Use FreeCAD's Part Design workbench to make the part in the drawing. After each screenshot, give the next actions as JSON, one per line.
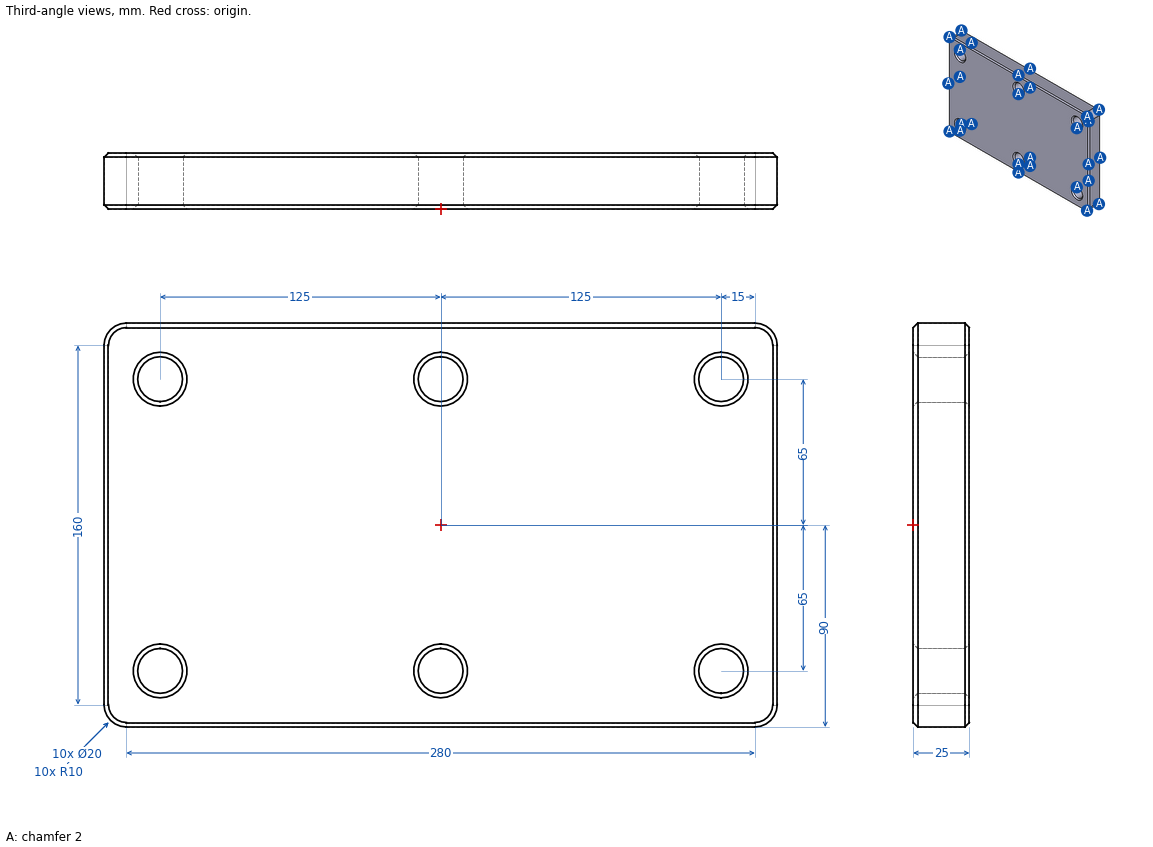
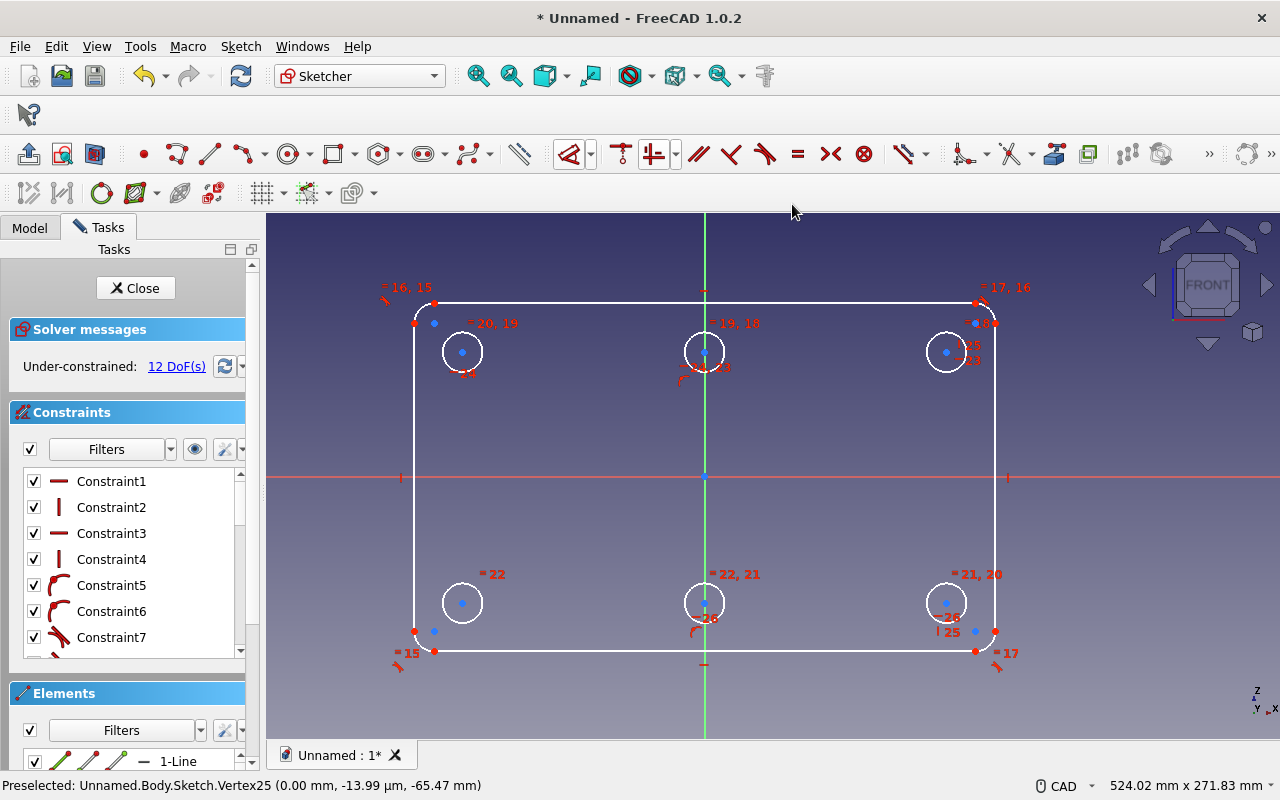
{"action": "left_click", "coordinate": [463, 352]}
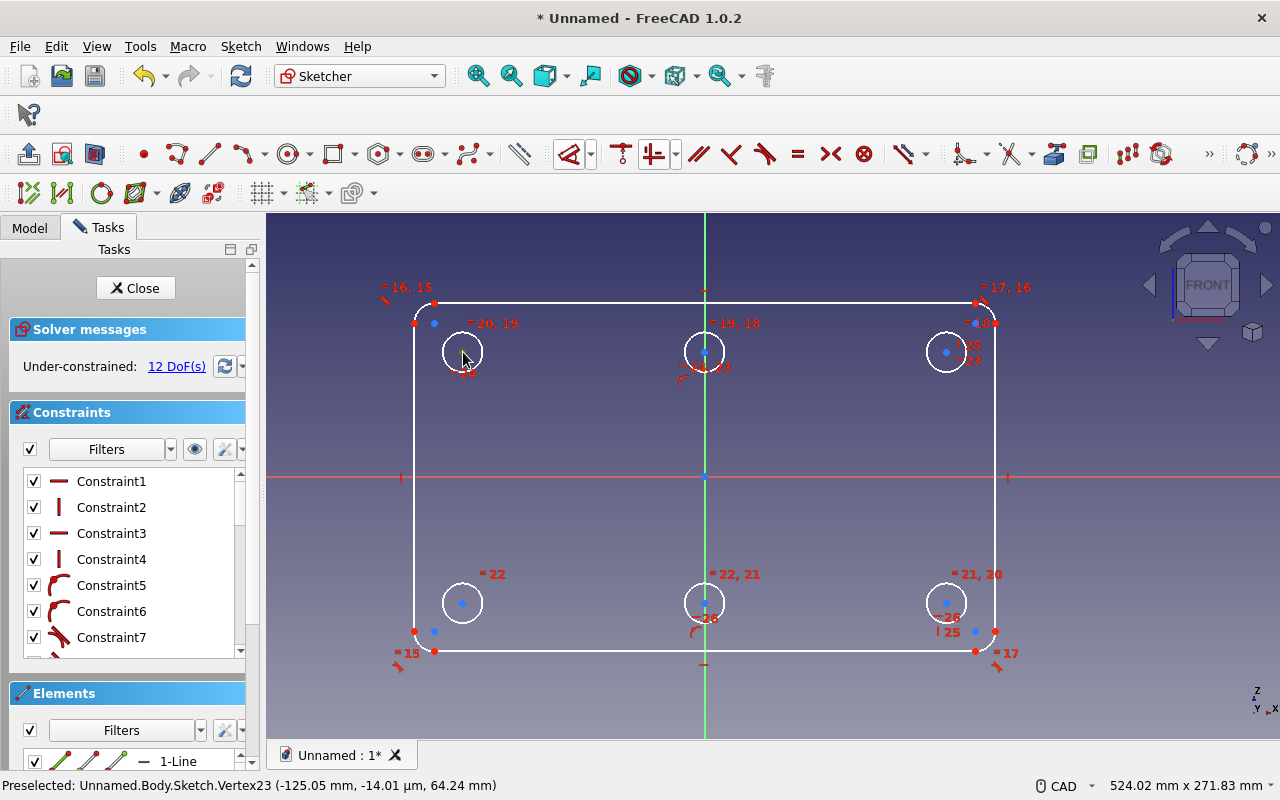
{"action": "left_click", "coordinate": [463, 603]}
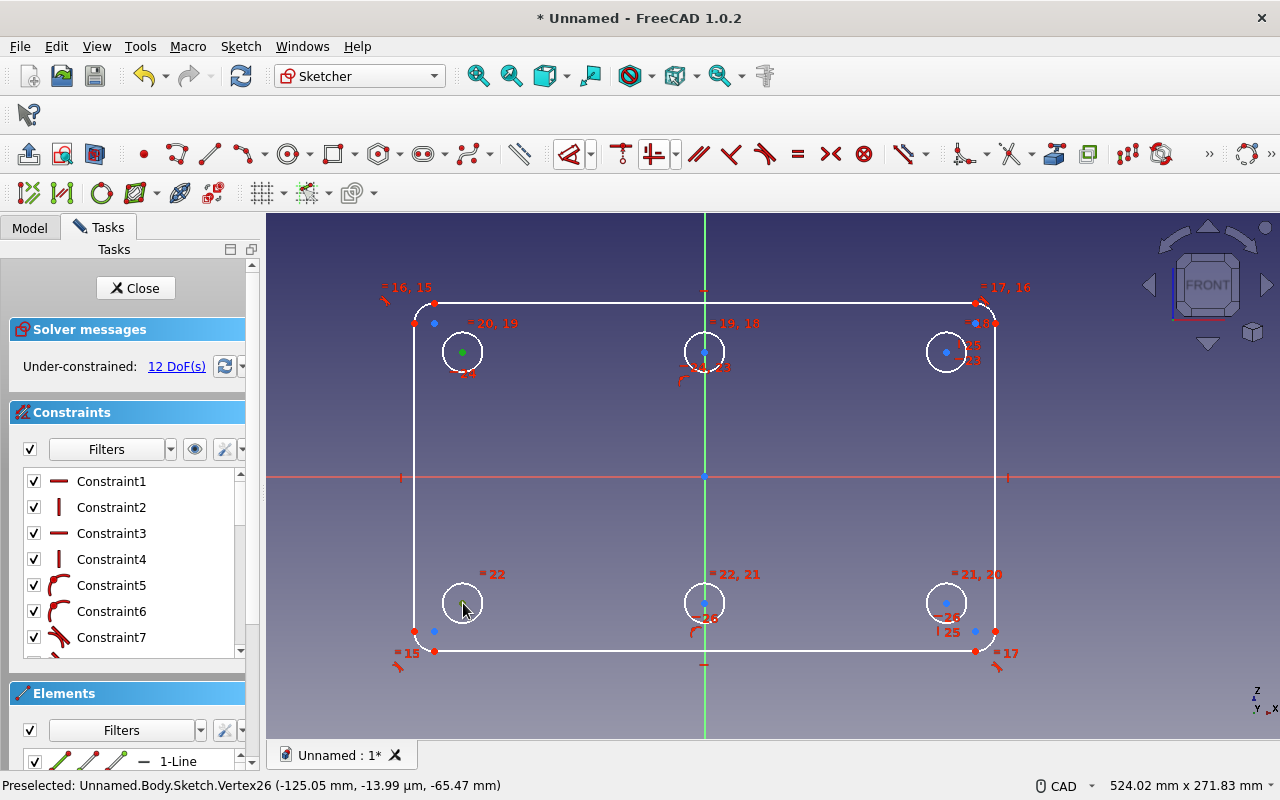
{"action": "left_click", "coordinate": [676, 154]}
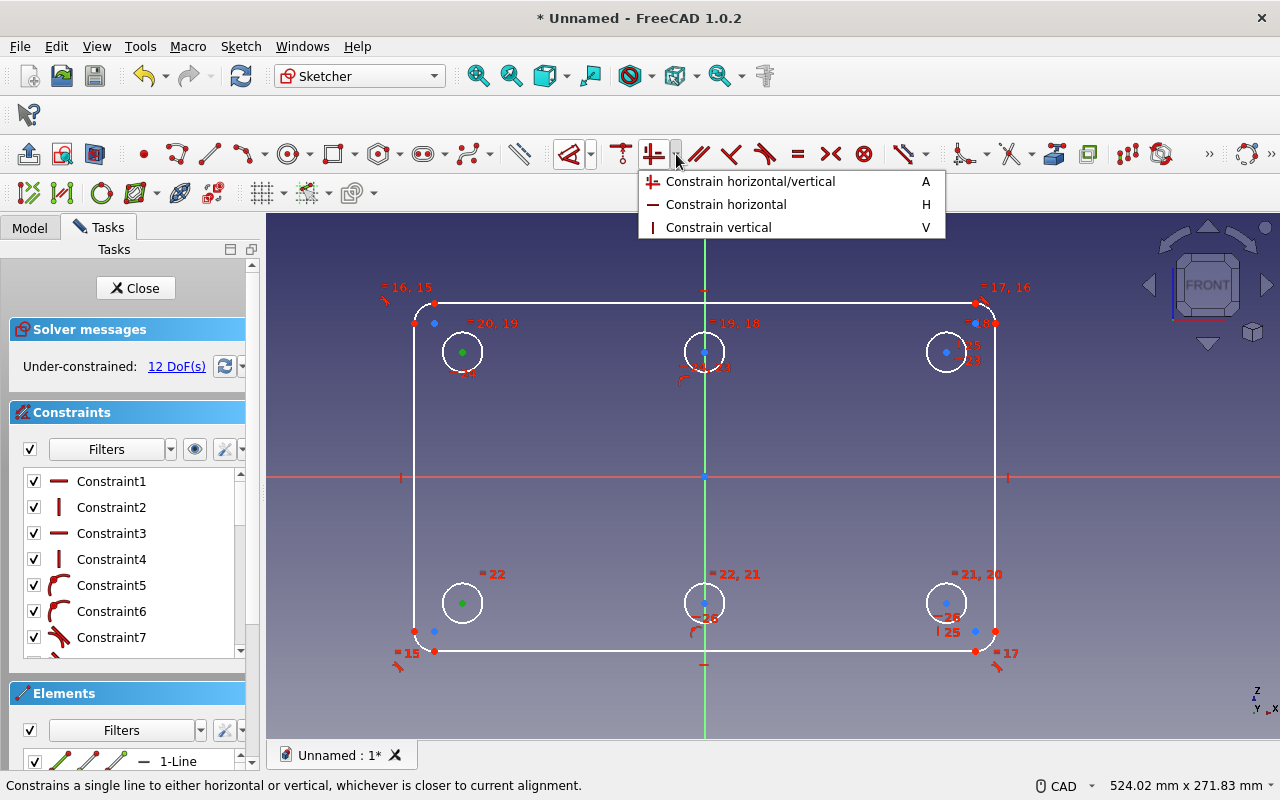
{"action": "left_click", "coordinate": [792, 228]}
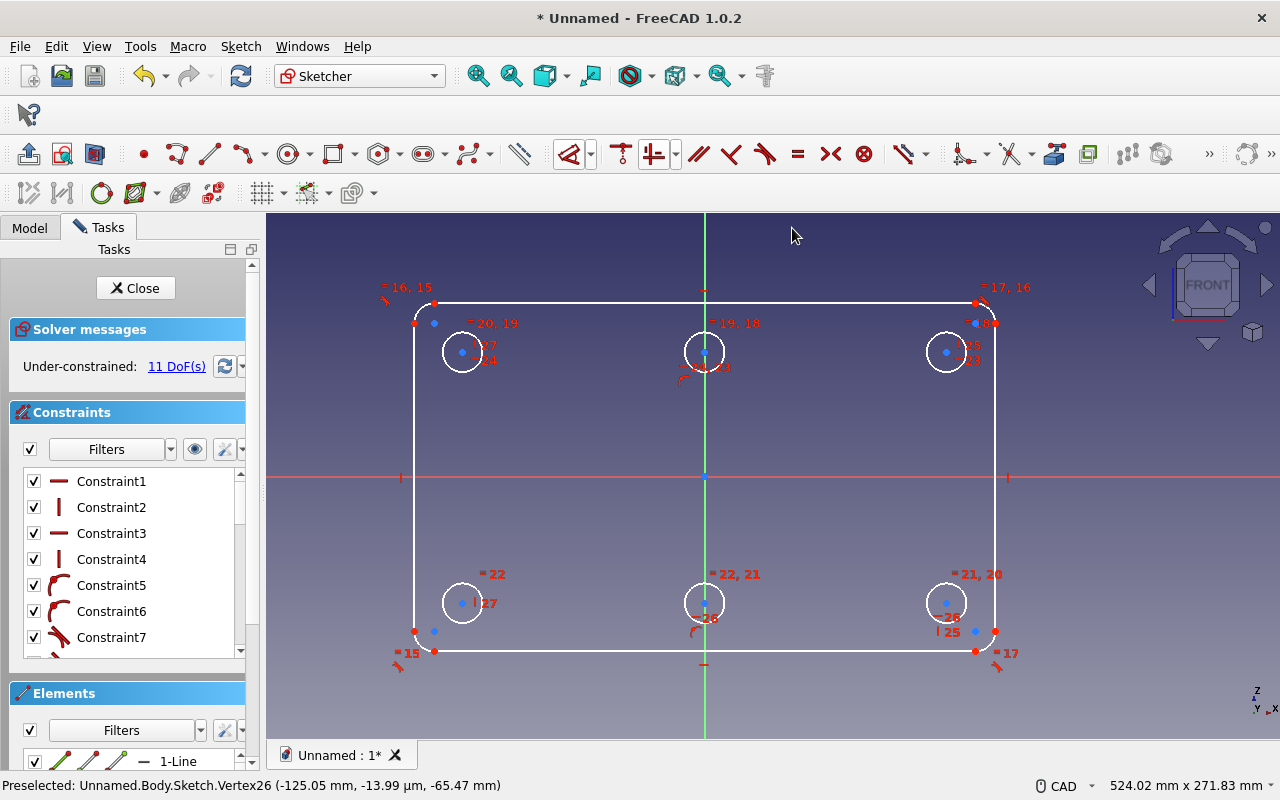
{"action": "left_click", "coordinate": [705, 603]}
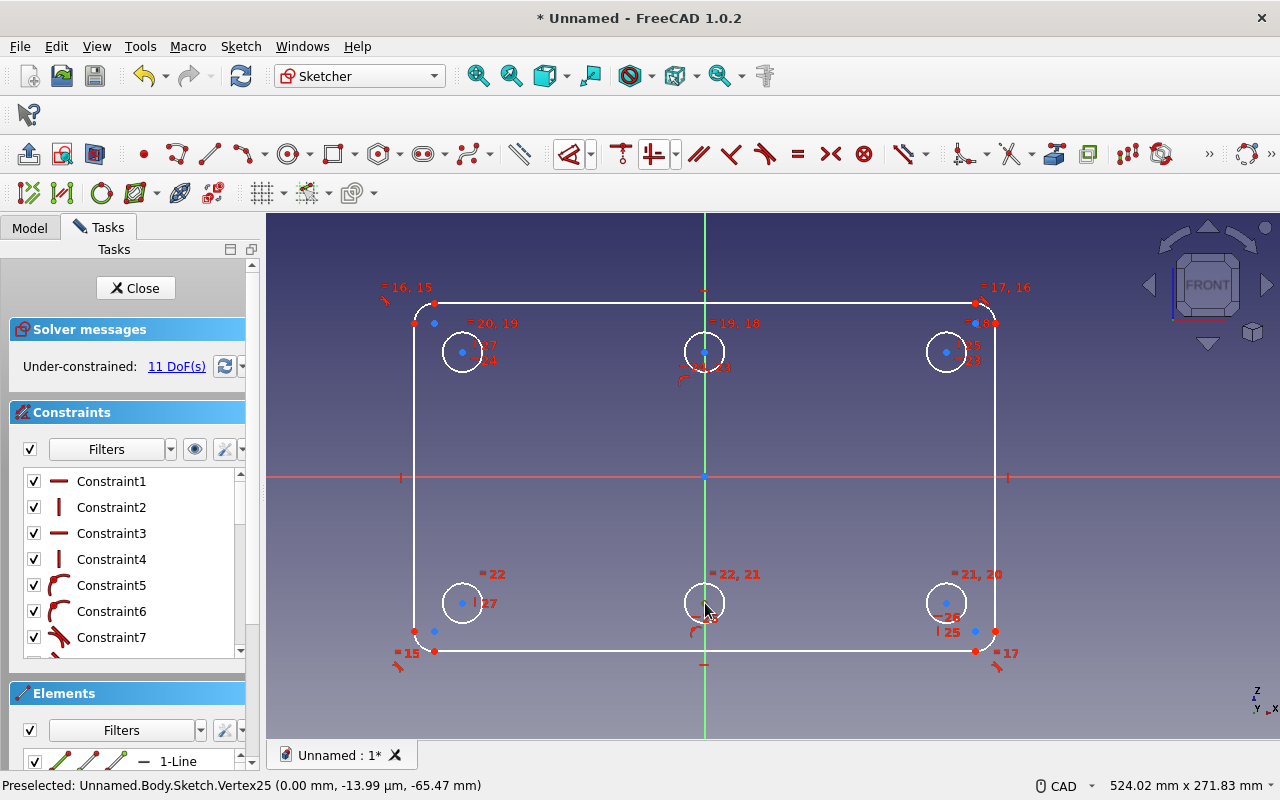
{"action": "left_click", "coordinate": [463, 603]}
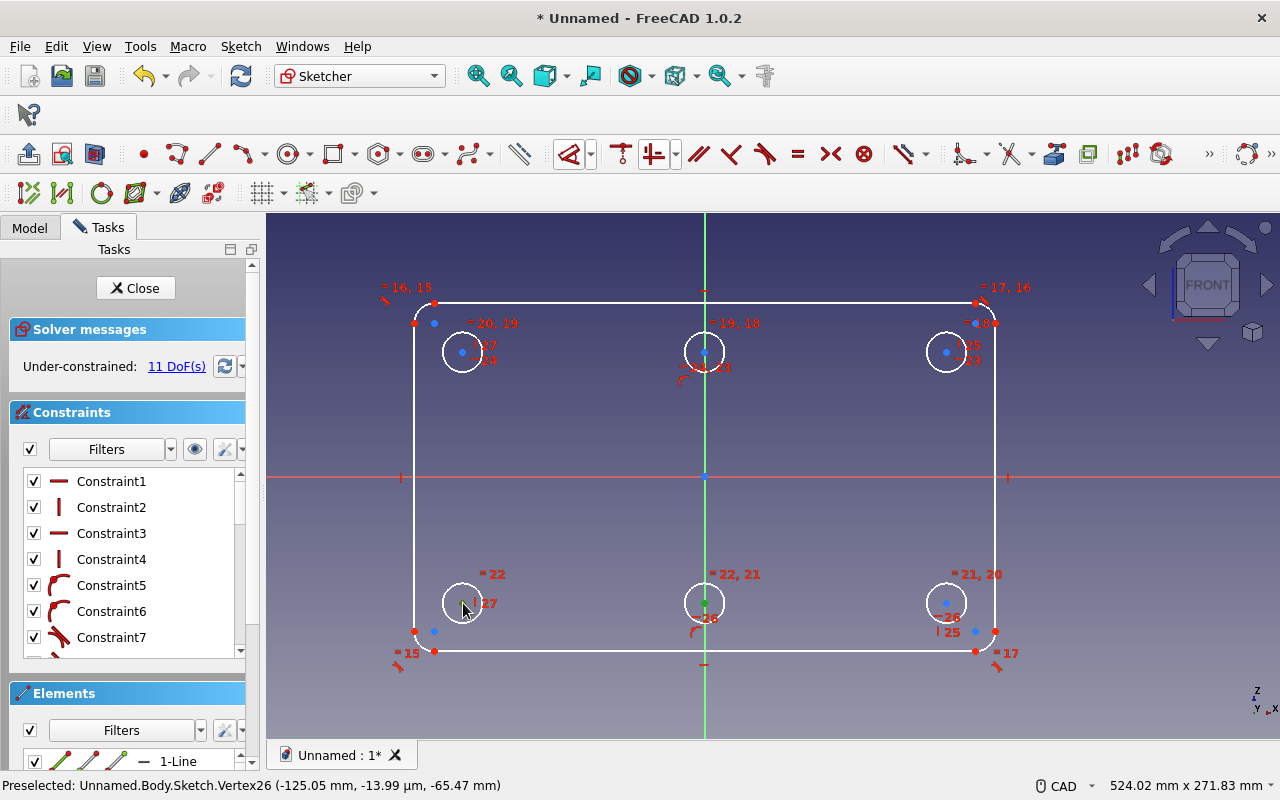
{"action": "key", "text": "h"}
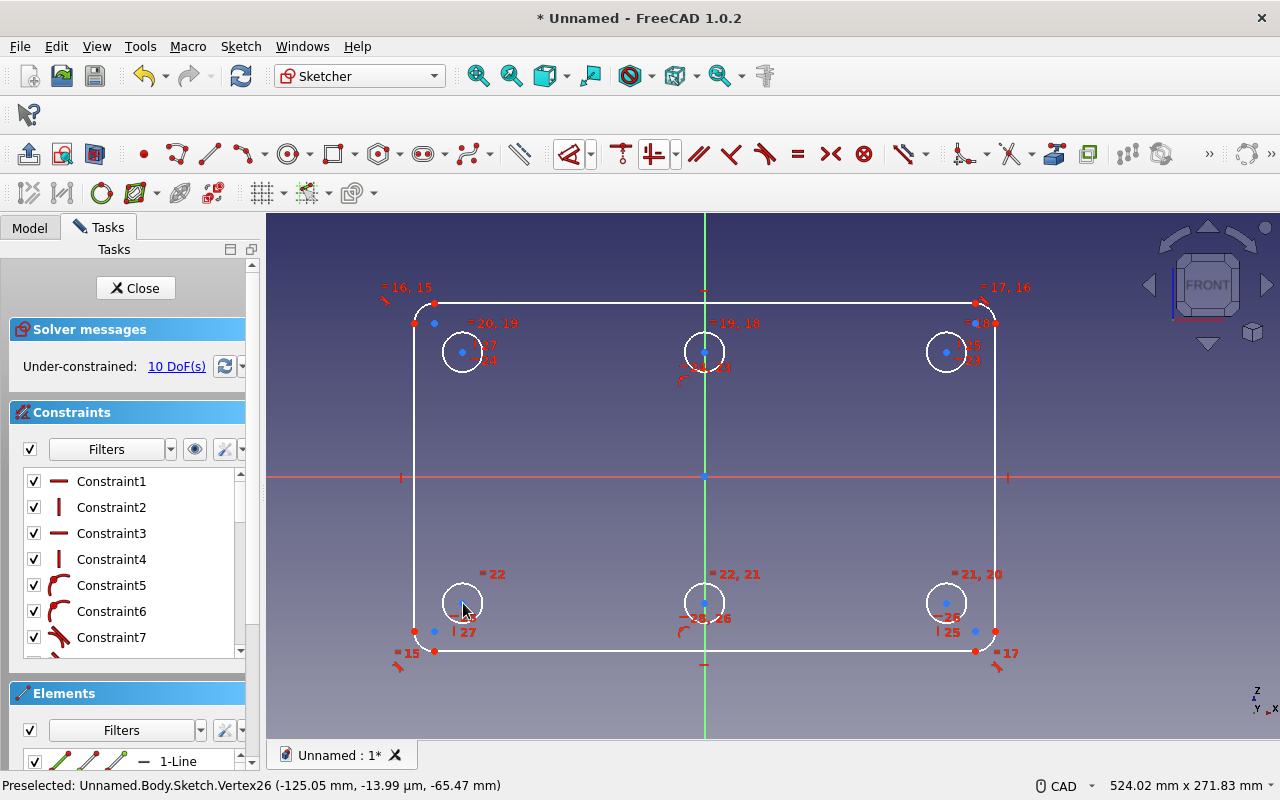
{"action": "scroll", "coordinate": [416, 641], "scroll_direction": "up", "scroll_amount": 4}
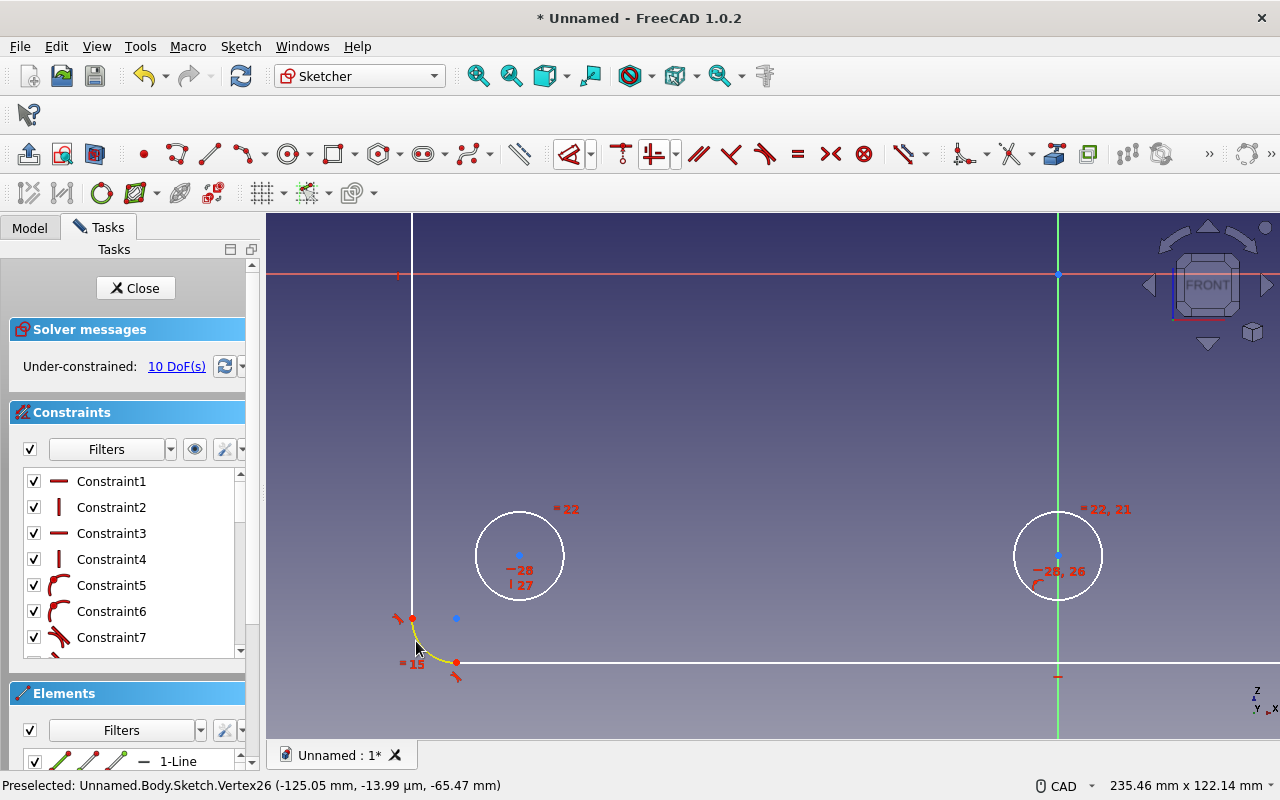
{"action": "left_click", "coordinate": [417, 639]}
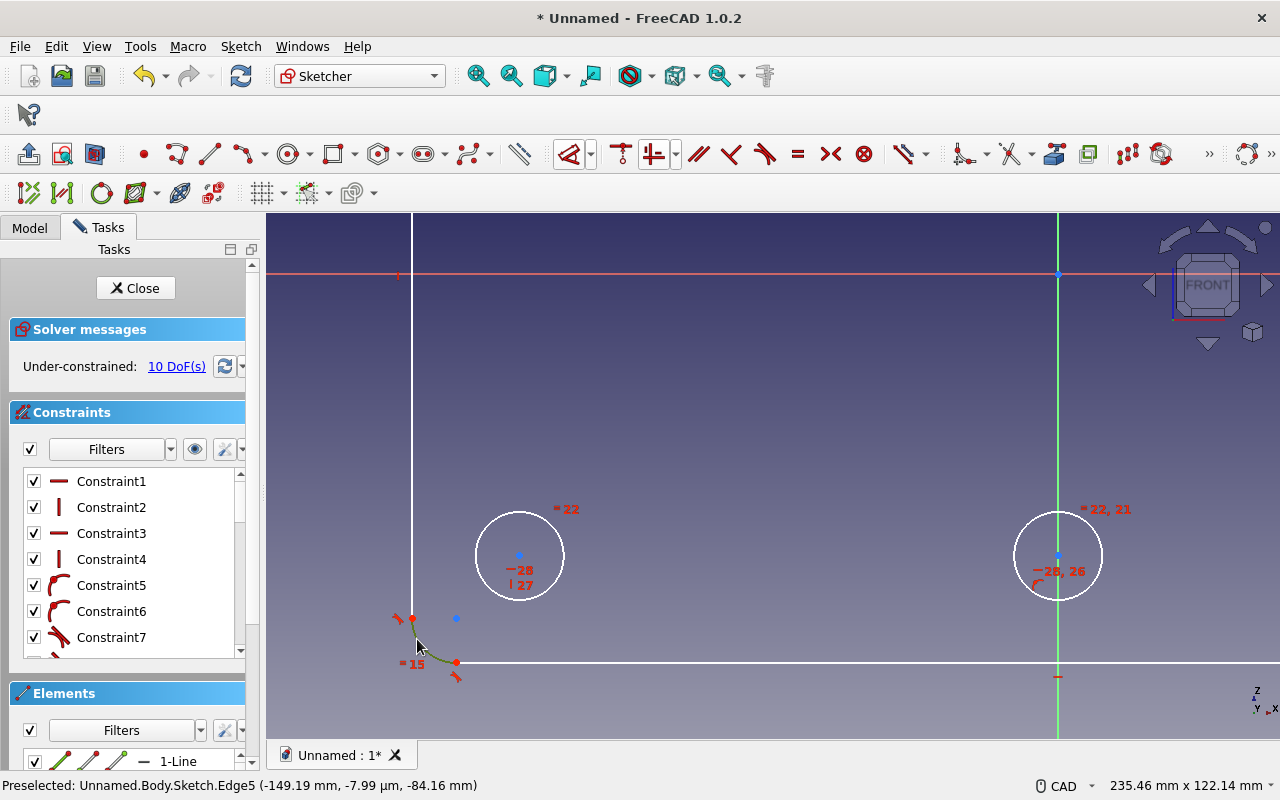
{"action": "left_click", "coordinate": [590, 154]}